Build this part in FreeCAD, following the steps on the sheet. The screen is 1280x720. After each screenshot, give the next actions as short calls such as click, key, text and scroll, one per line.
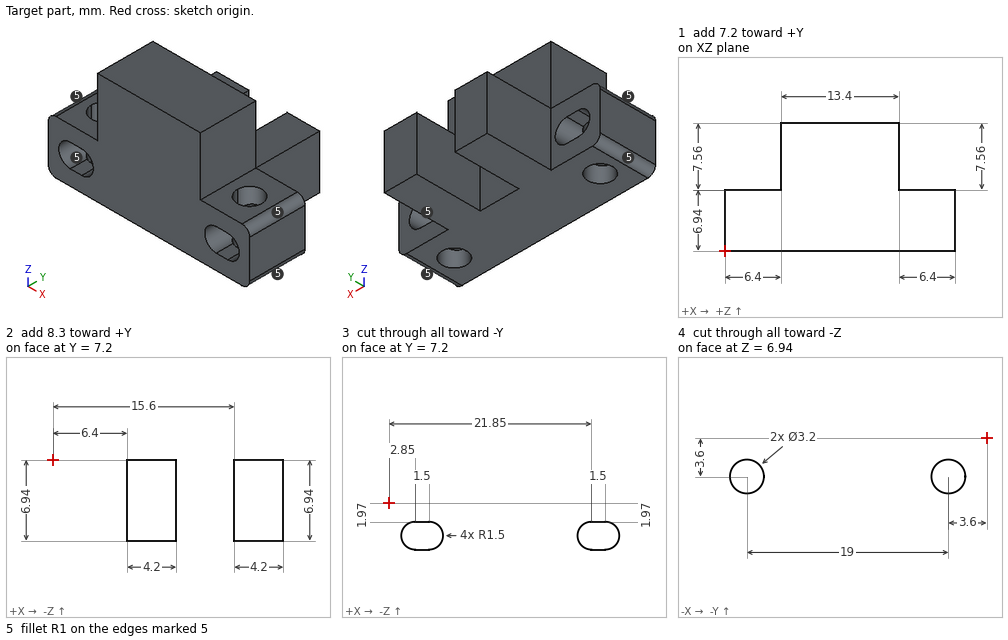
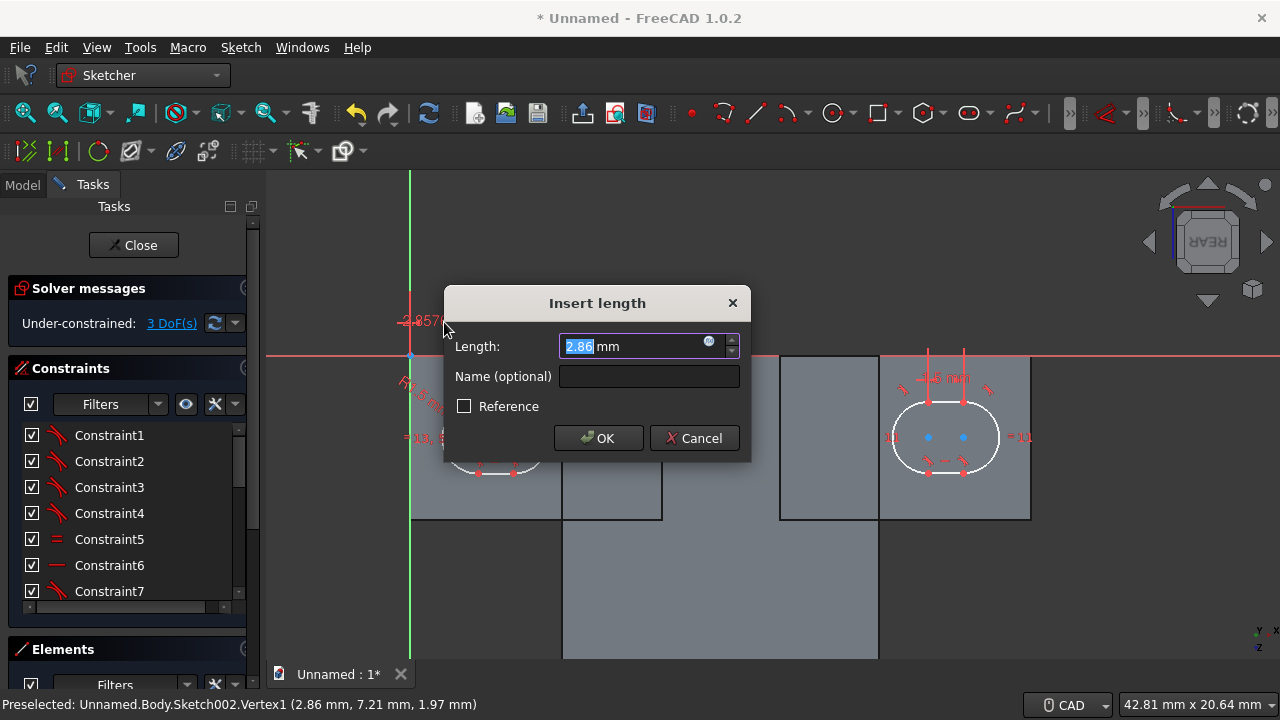
text(2.85)
key(Return)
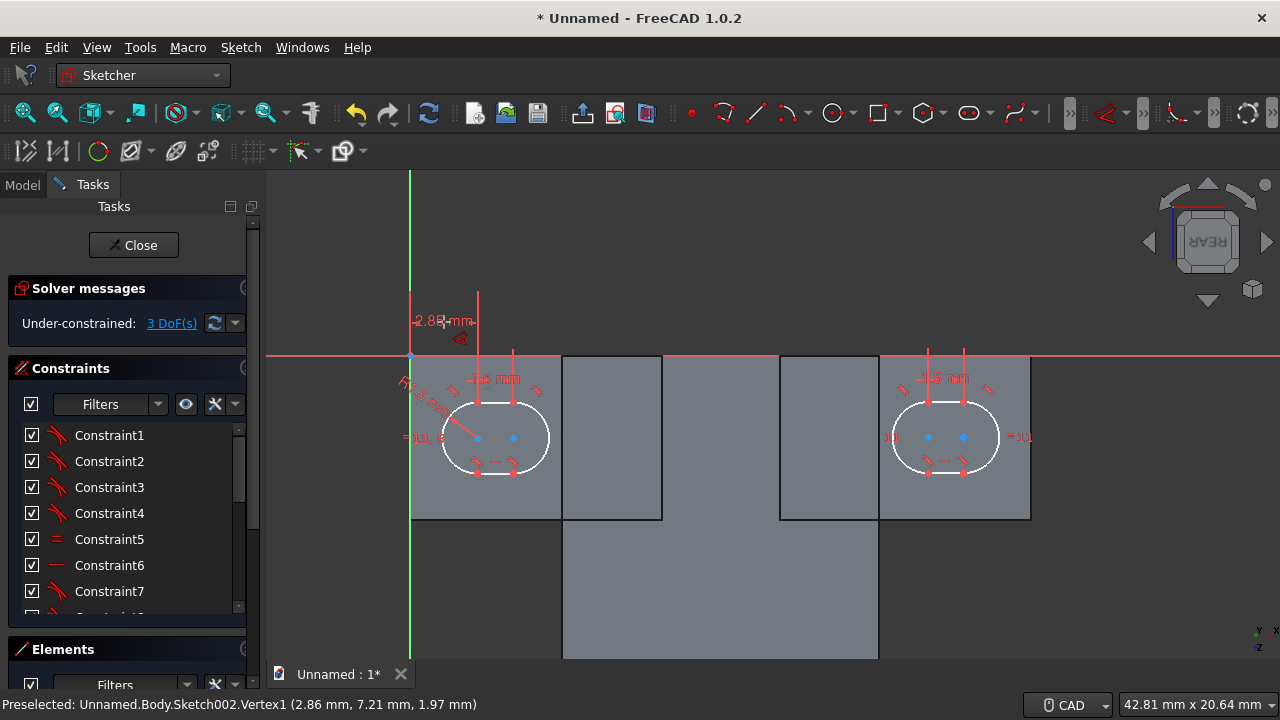
click(478, 403)
click(352, 379)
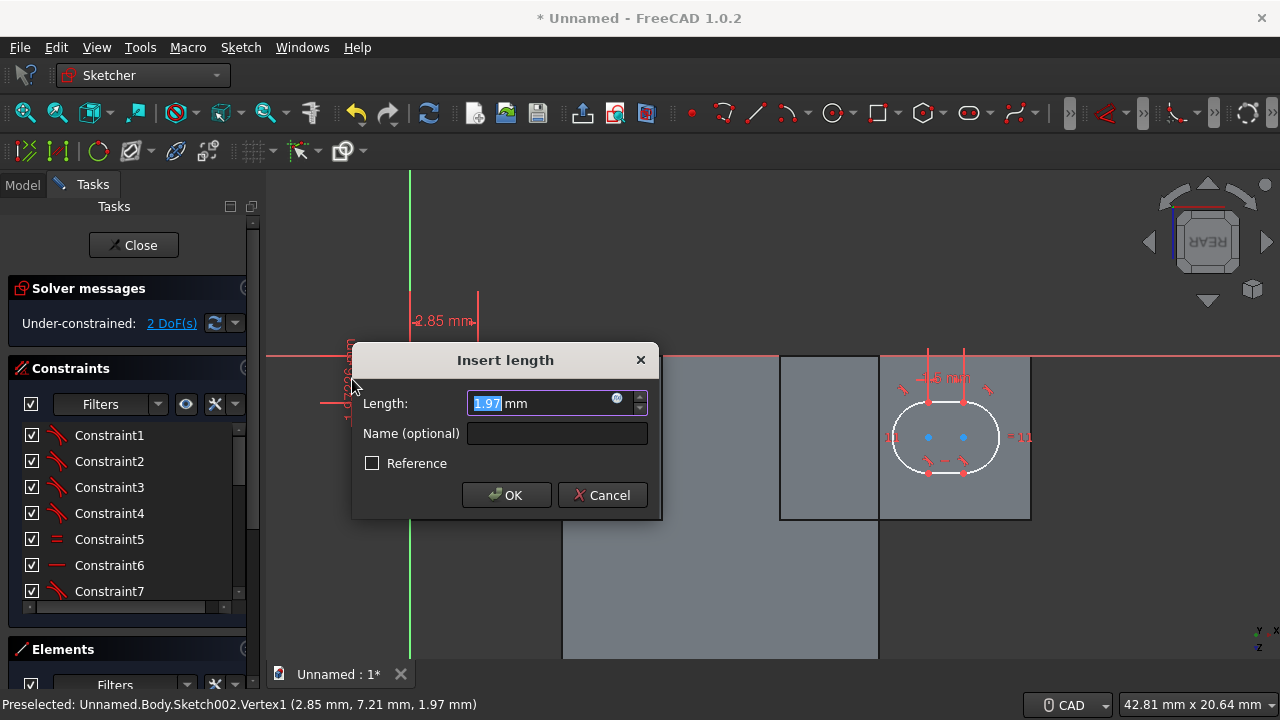
text(1.97)
key(Return)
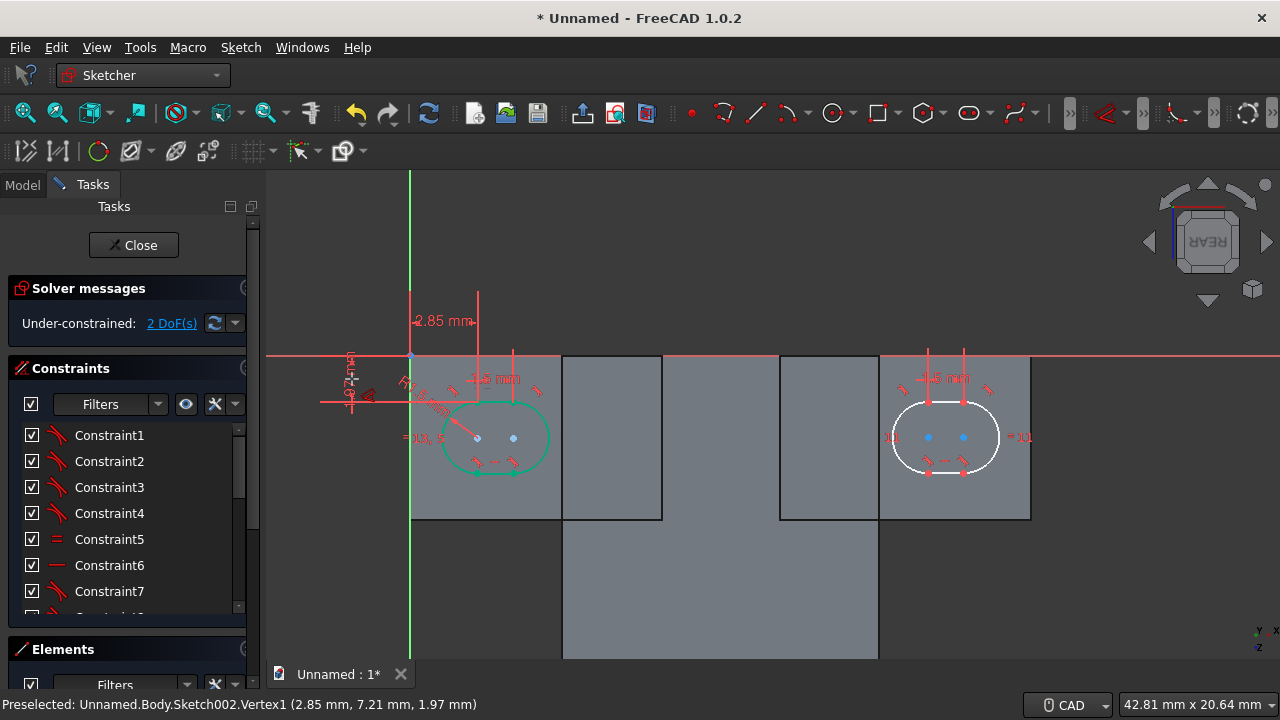
click(928, 402)
click(1034, 379)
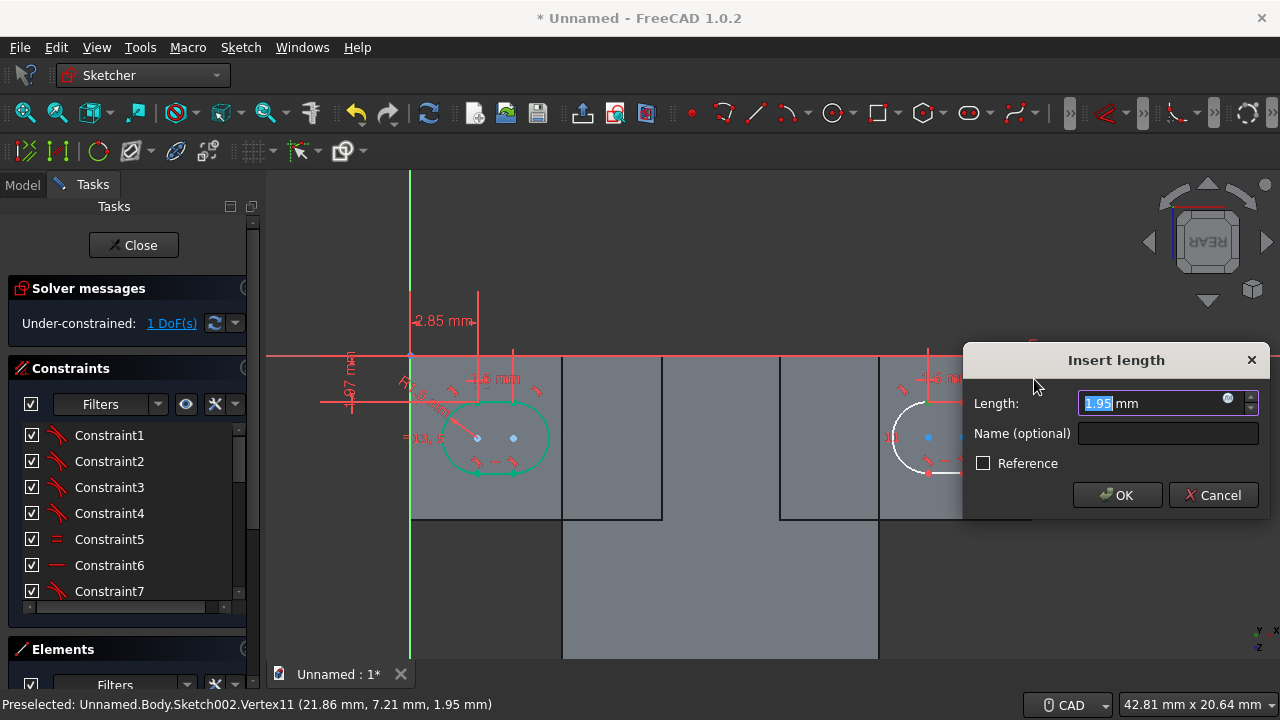
text(1.97)
key(Return)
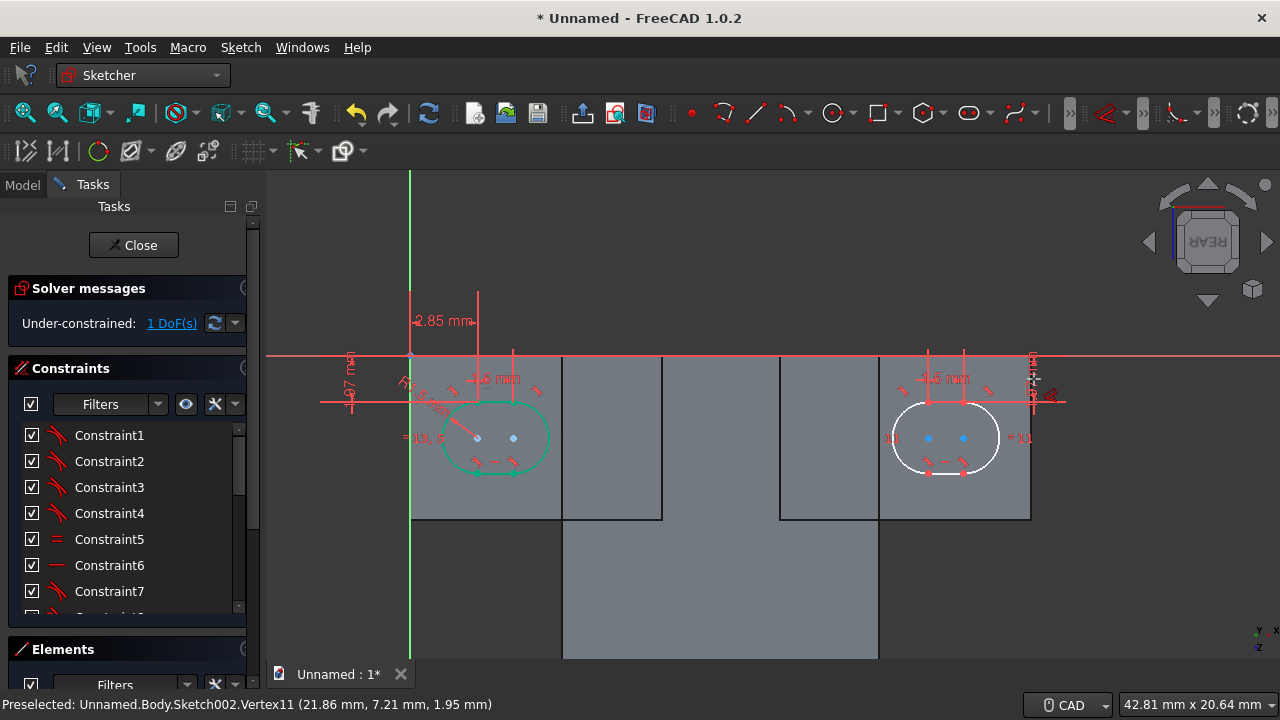
click(928, 402)
click(669, 322)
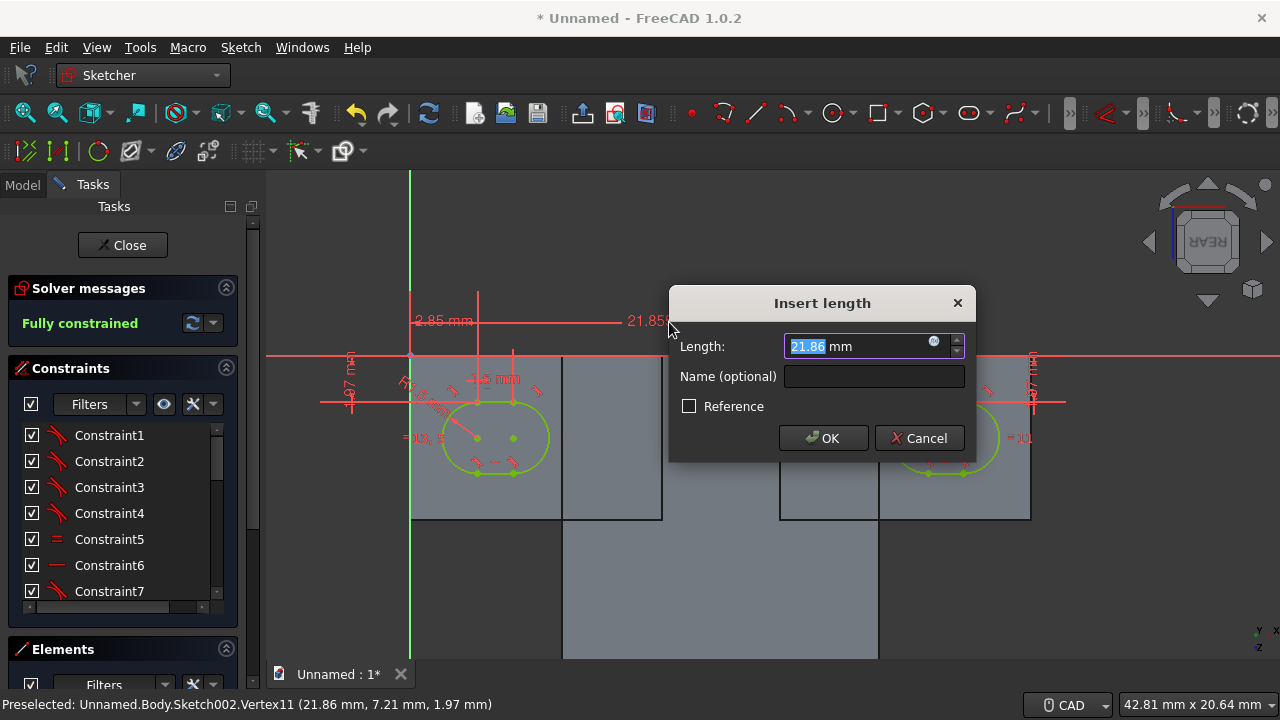
text(21.85)
key(Return)
key(Escape)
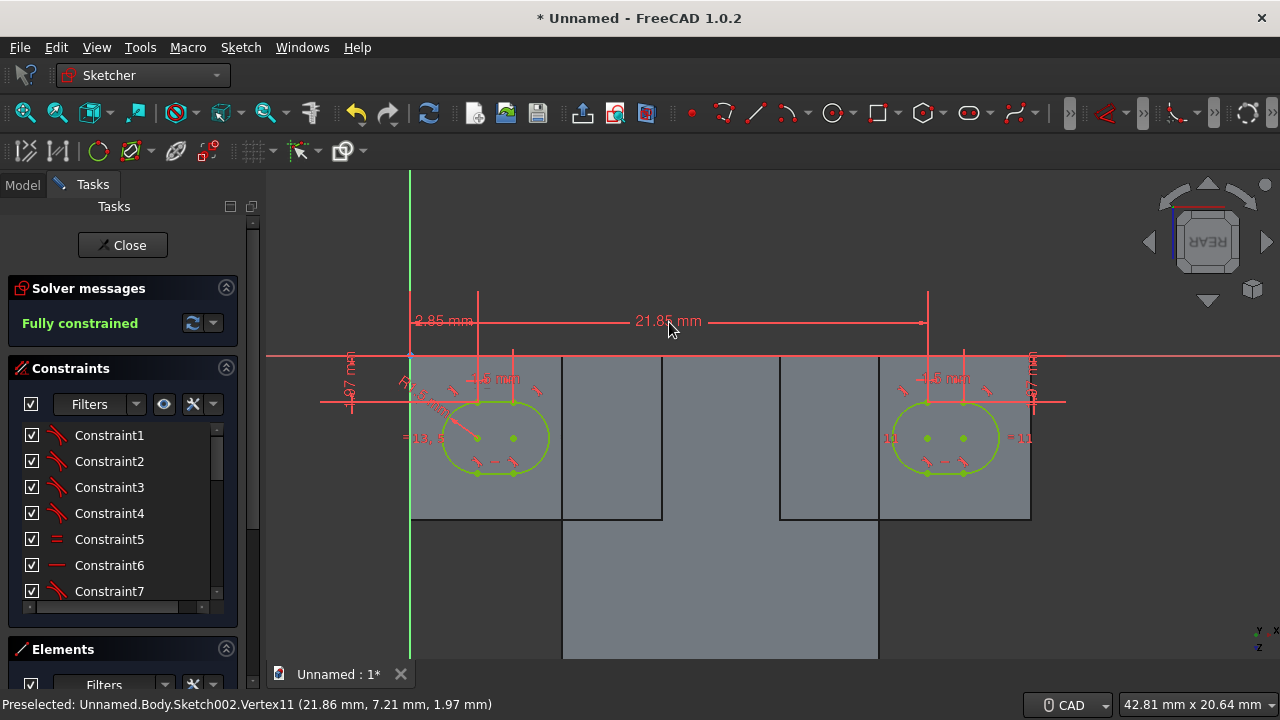
click(123, 245)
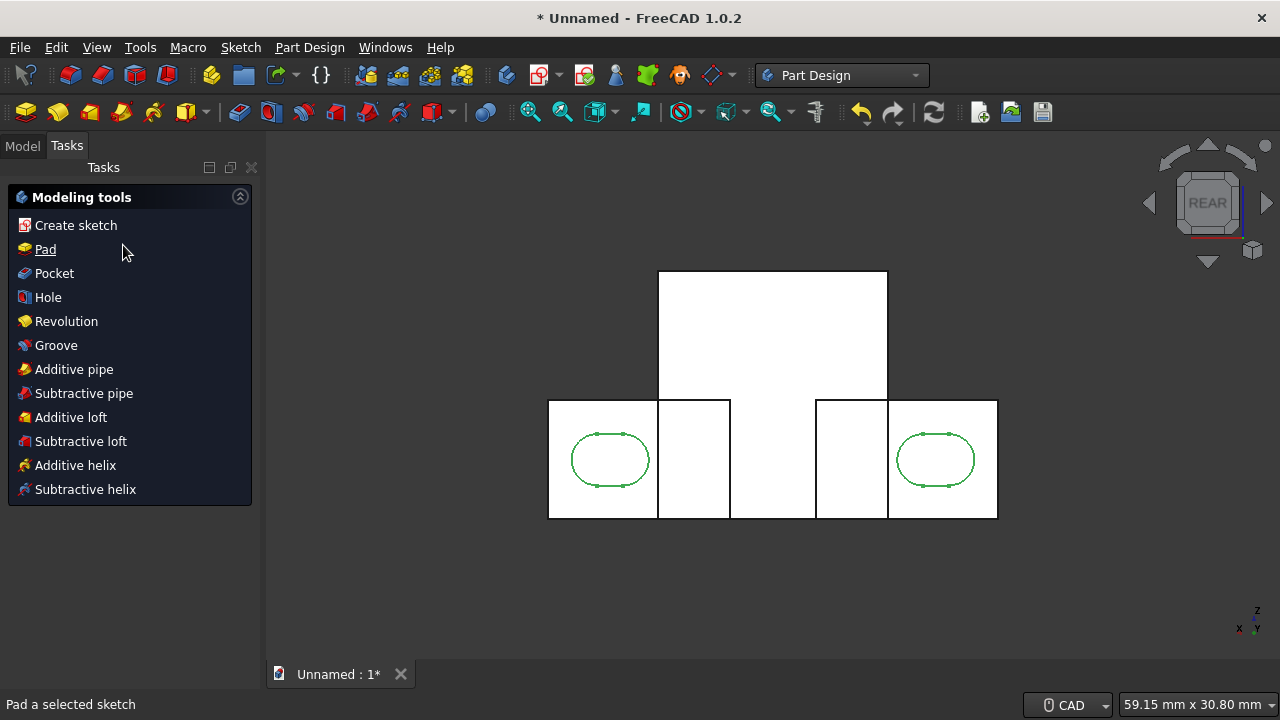
click(240, 112)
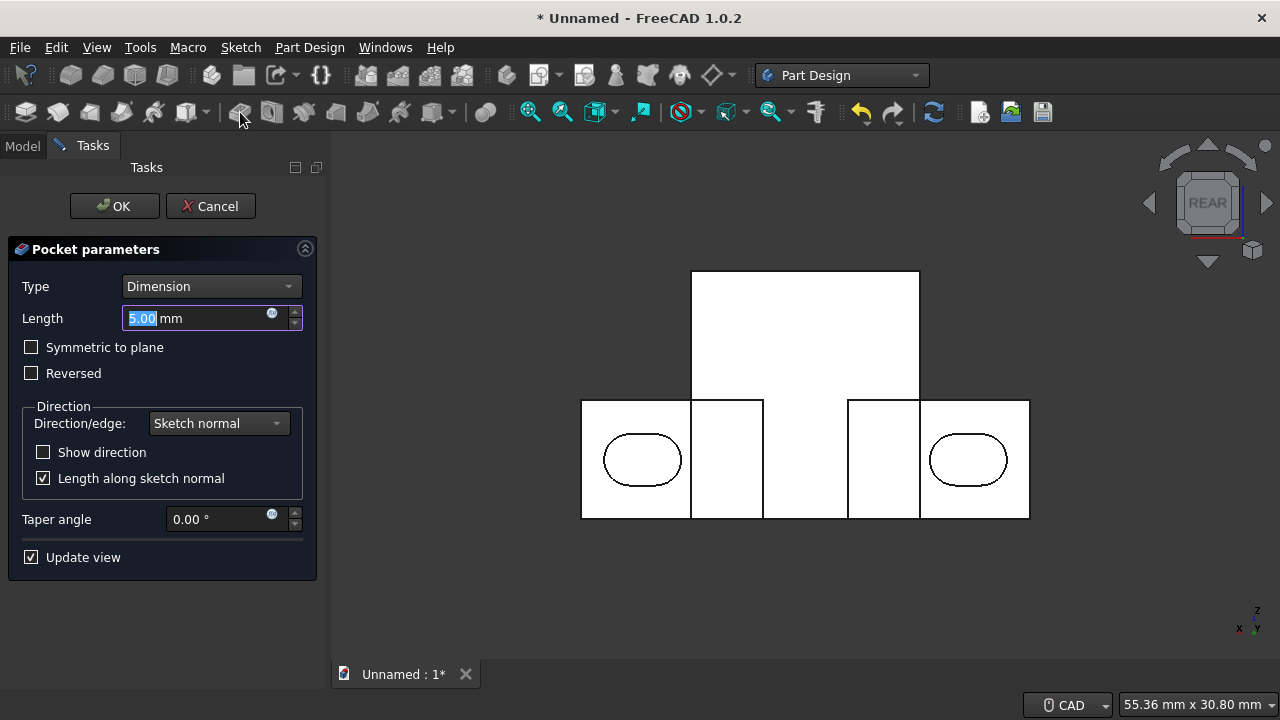
click(212, 286)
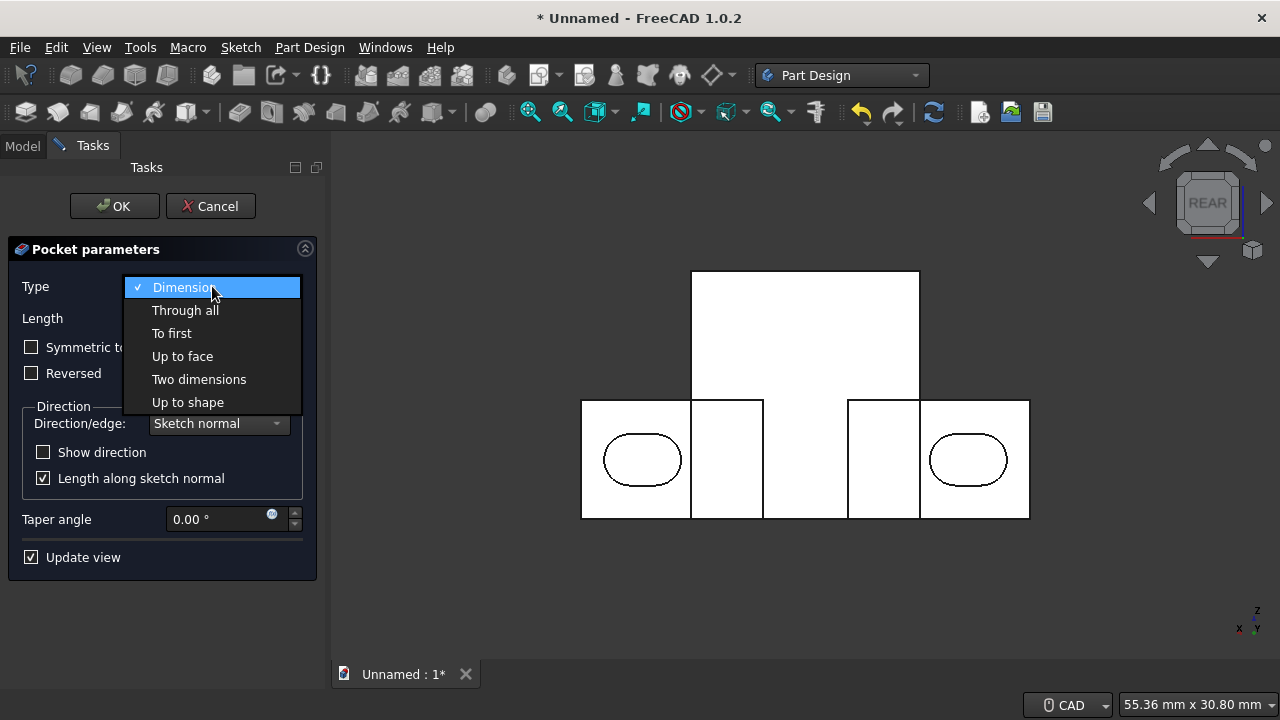
click(212, 310)